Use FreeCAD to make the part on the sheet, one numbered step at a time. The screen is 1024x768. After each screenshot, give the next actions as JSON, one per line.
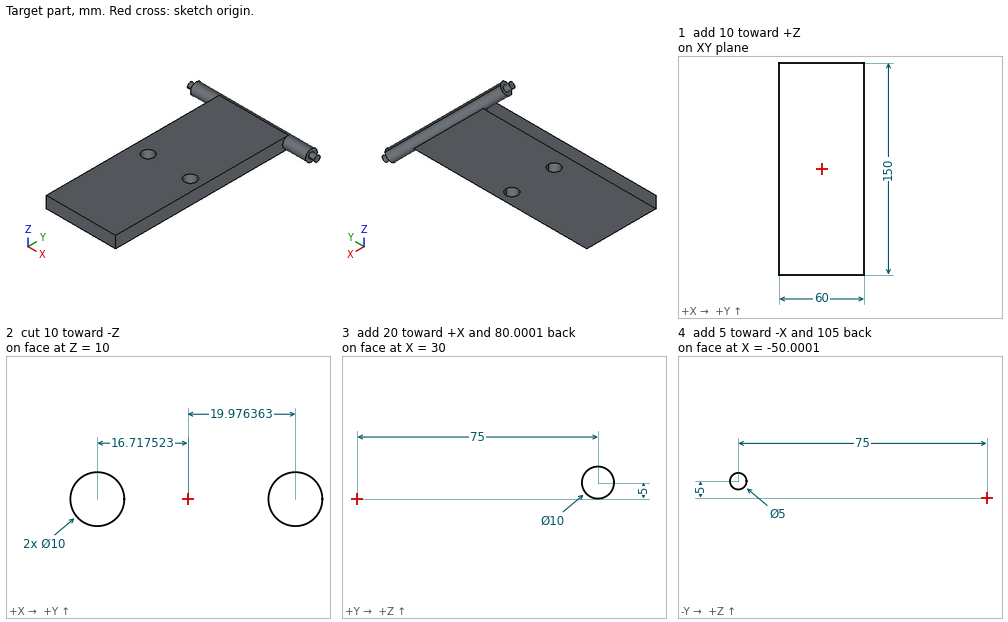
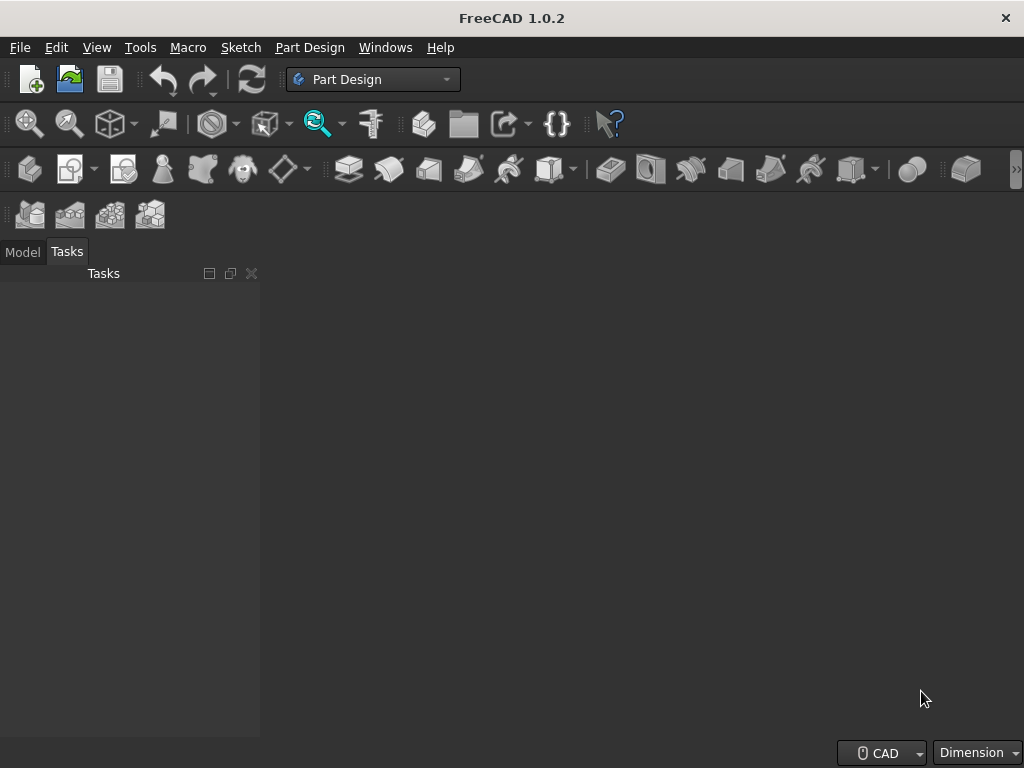
{"action": "left_click", "coordinate": [30, 80]}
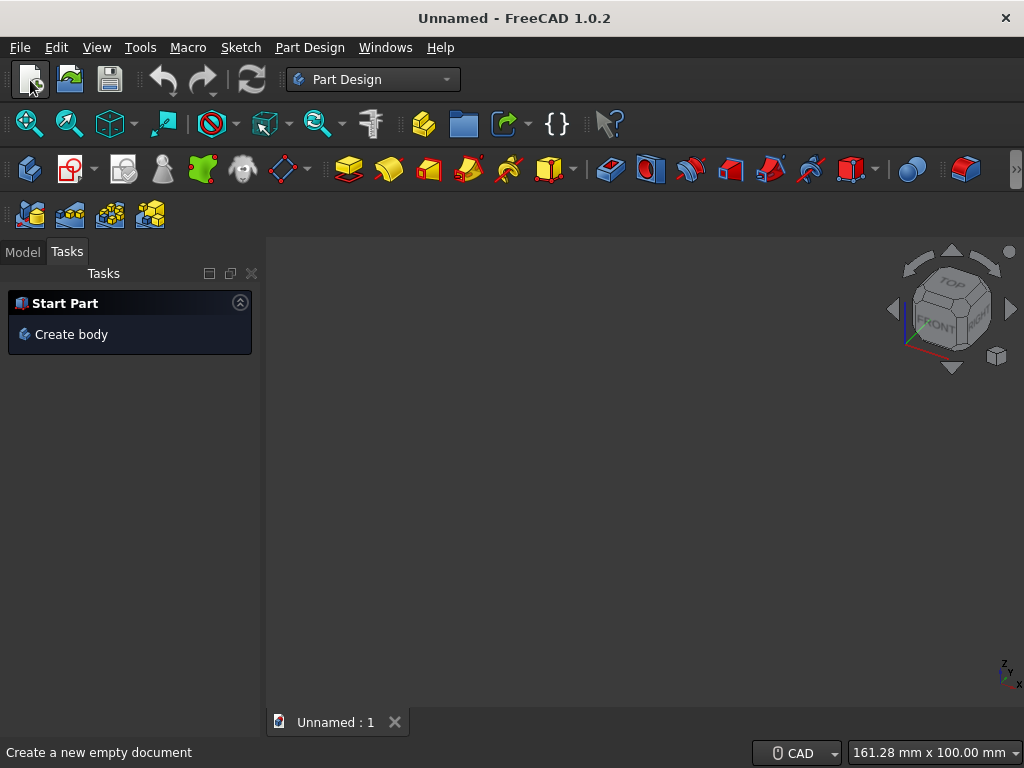
{"action": "left_click", "coordinate": [70, 170]}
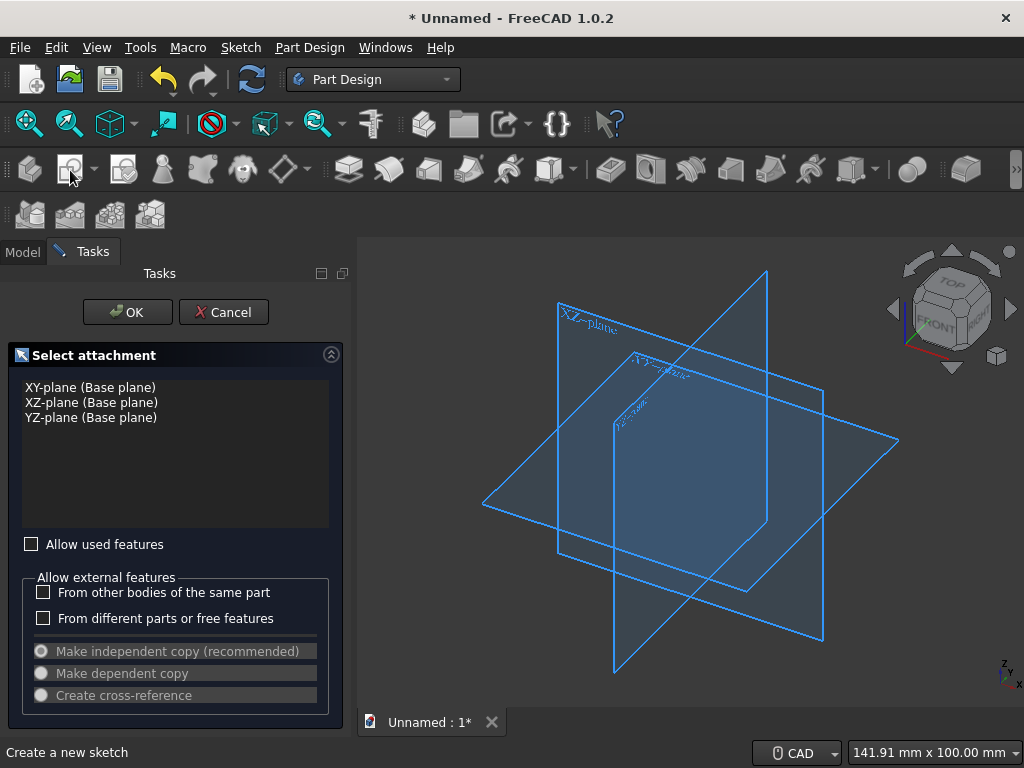
{"action": "left_click", "coordinate": [82, 388]}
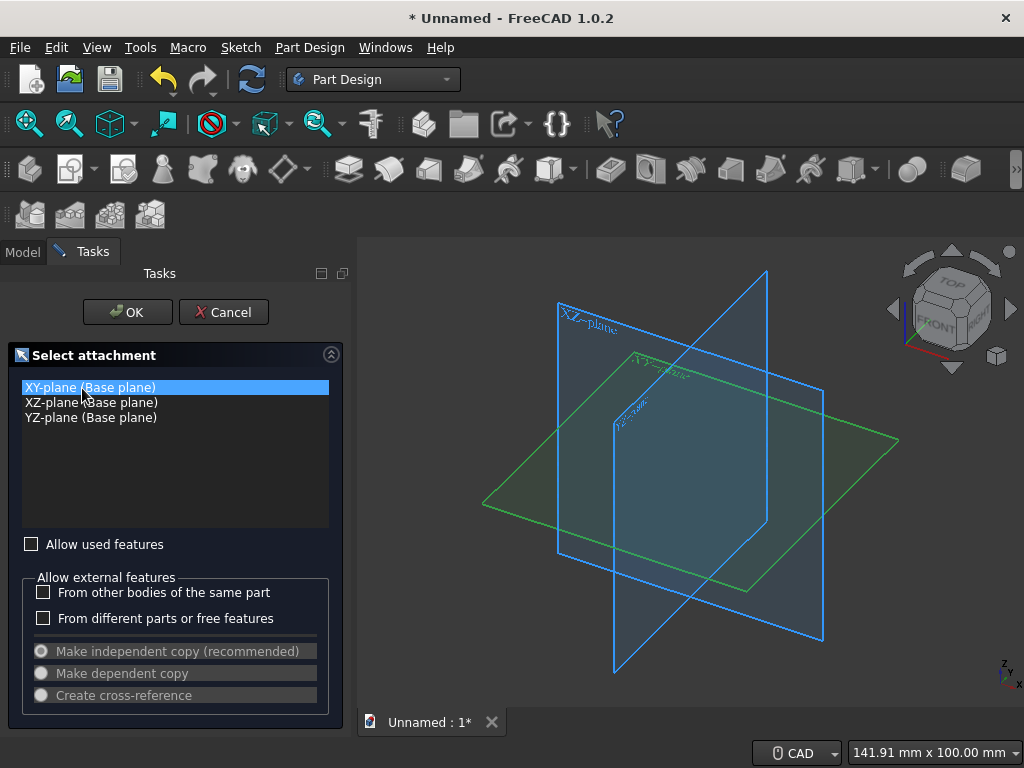
{"action": "left_click", "coordinate": [128, 312]}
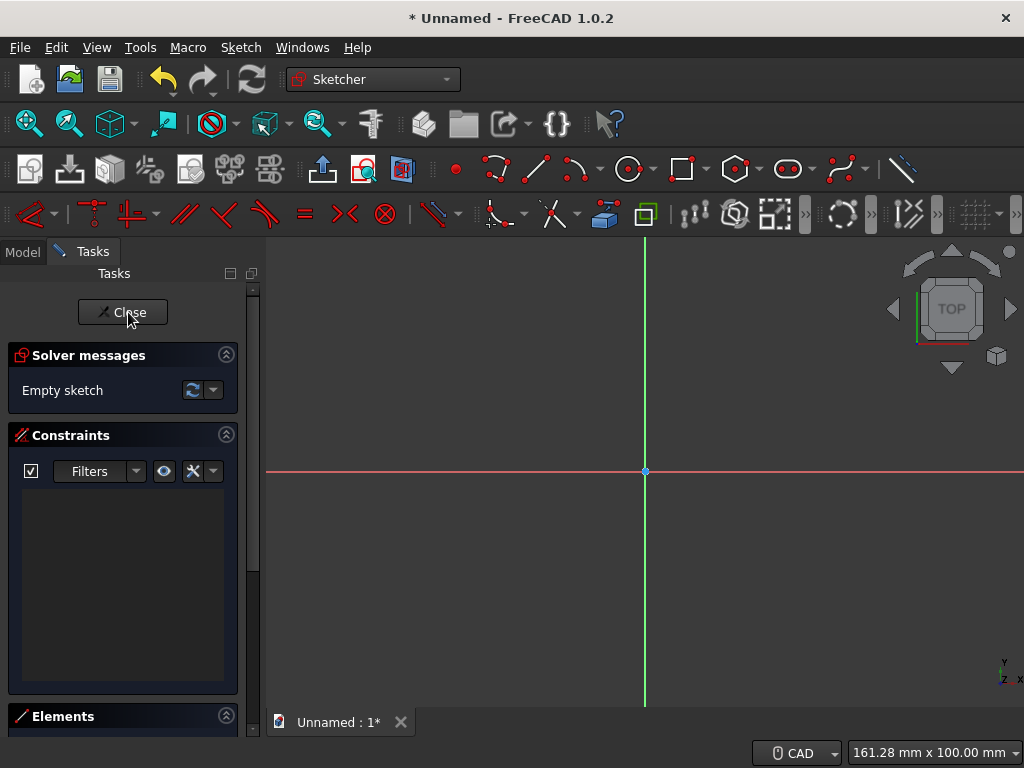
{"action": "scroll", "coordinate": [521, 472], "scroll_direction": "down", "scroll_amount": 4}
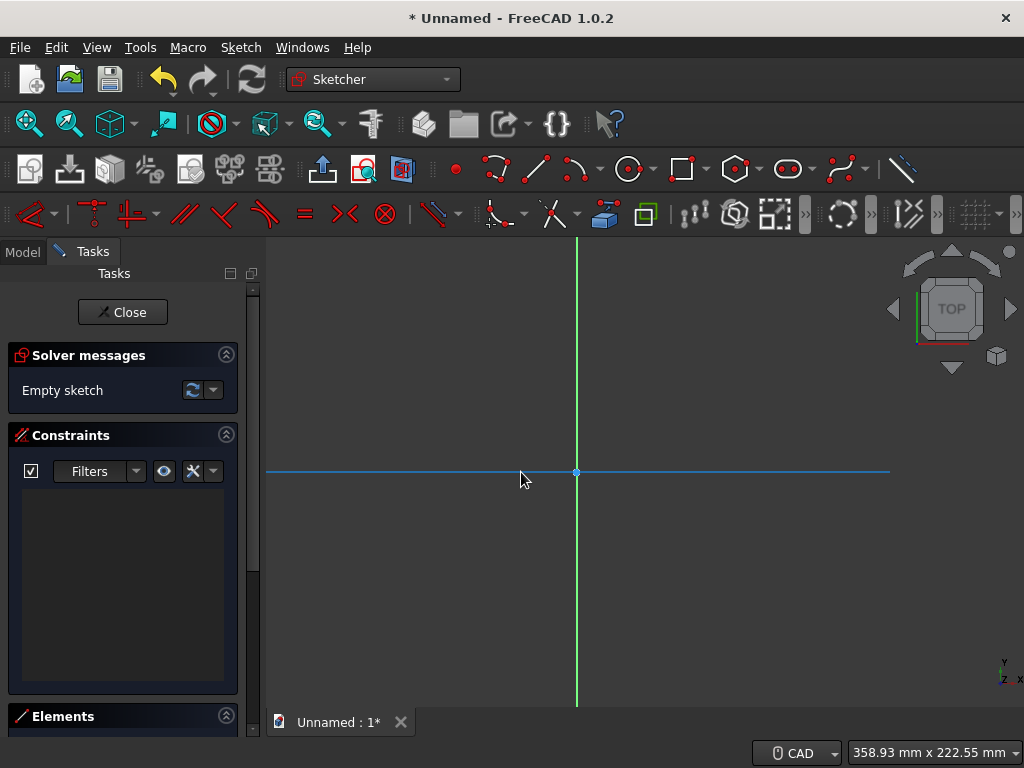
{"action": "left_click", "coordinate": [708, 170]}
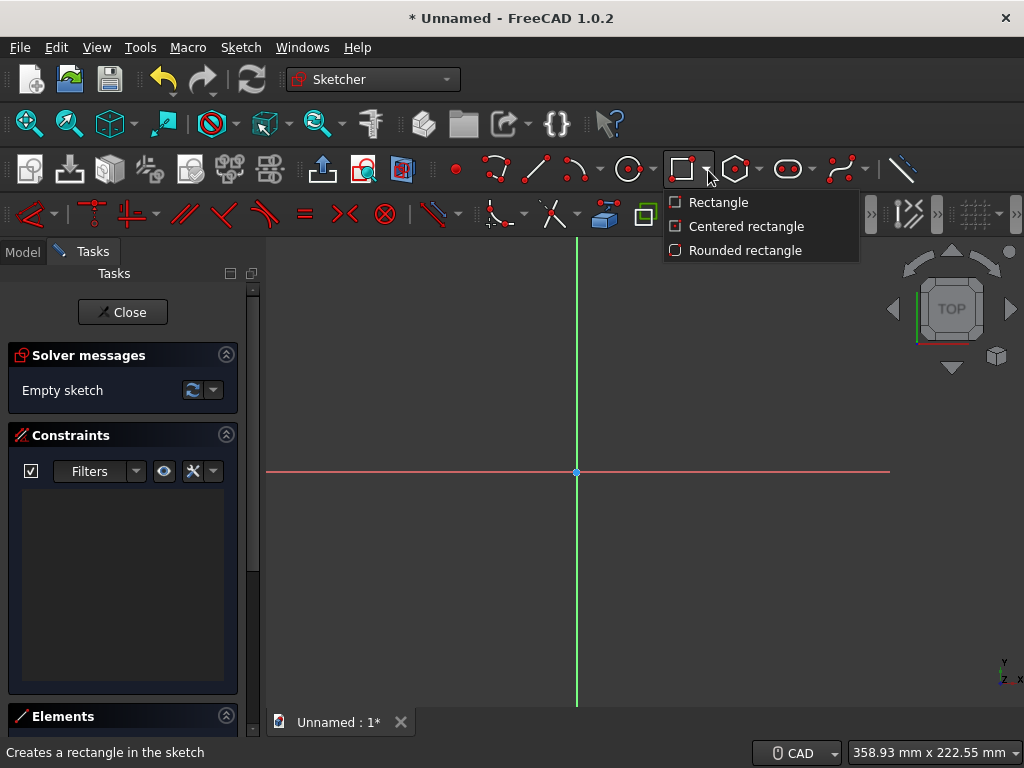
{"action": "left_click", "coordinate": [762, 226]}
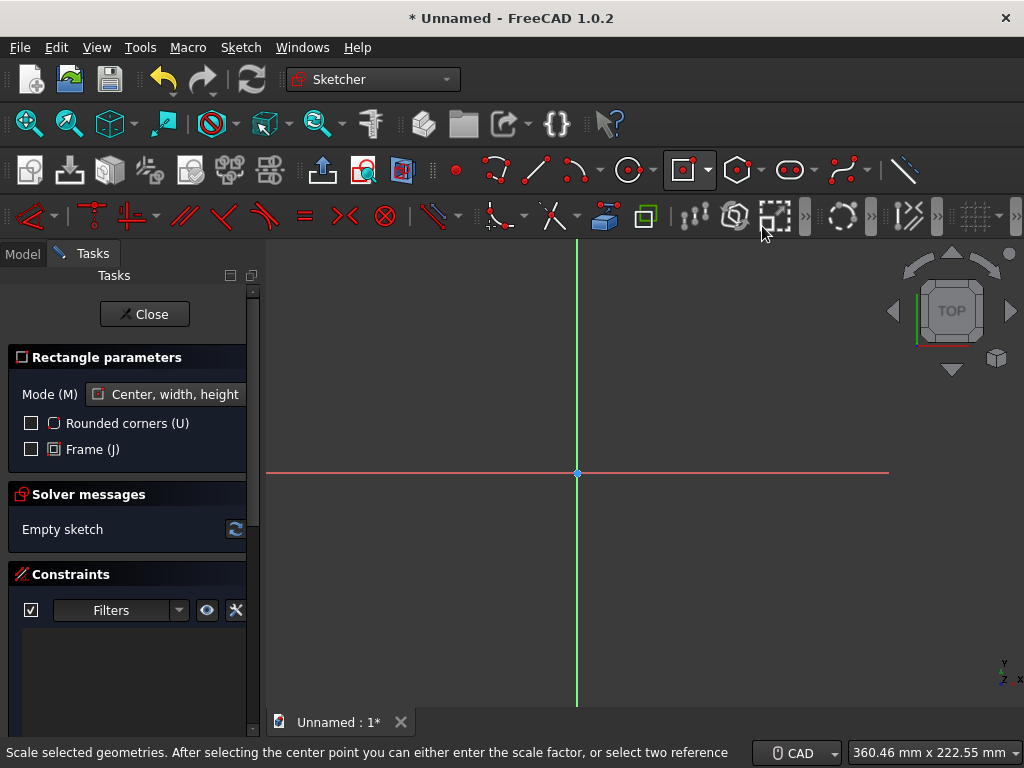
{"action": "left_click", "coordinate": [577, 473]}
{"action": "left_click", "coordinate": [640, 316]}
{"action": "key", "text": "Escape"}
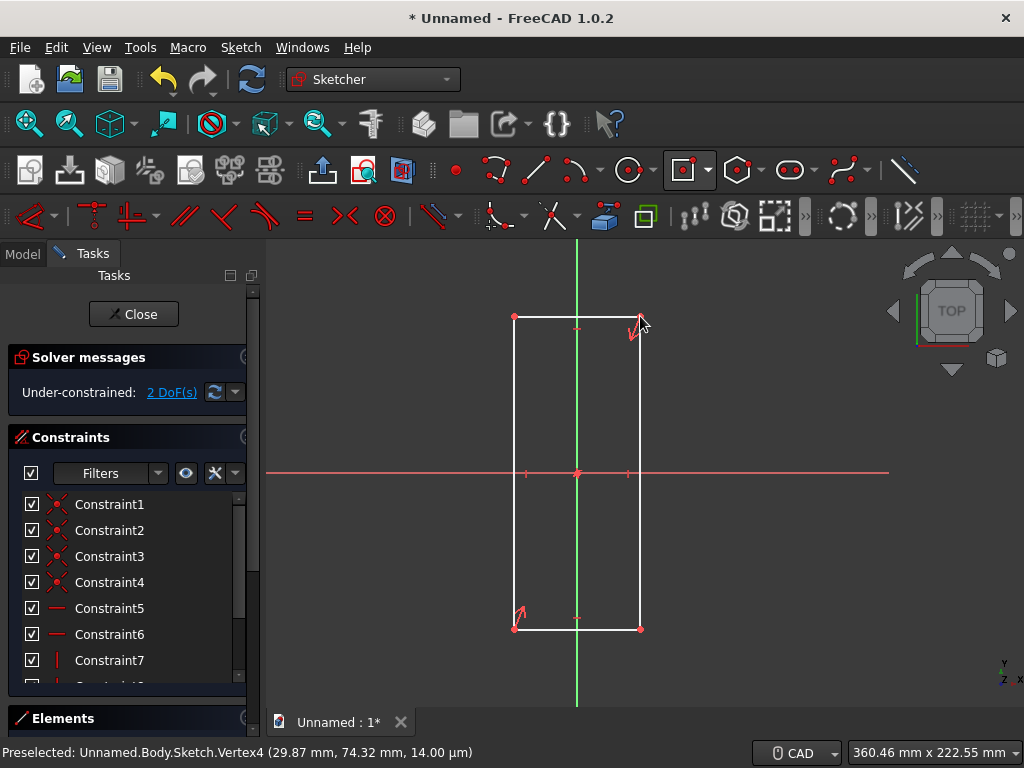
{"action": "left_click", "coordinate": [30, 216]}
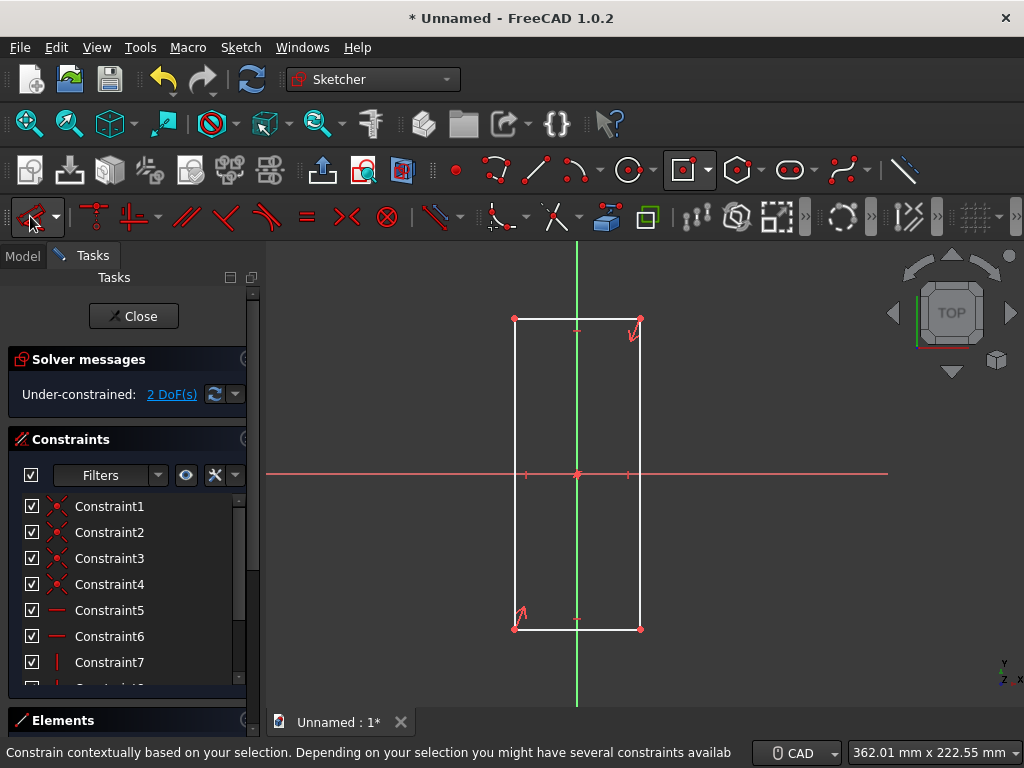
{"action": "left_click", "coordinate": [552, 630]}
{"action": "left_click", "coordinate": [549, 664]}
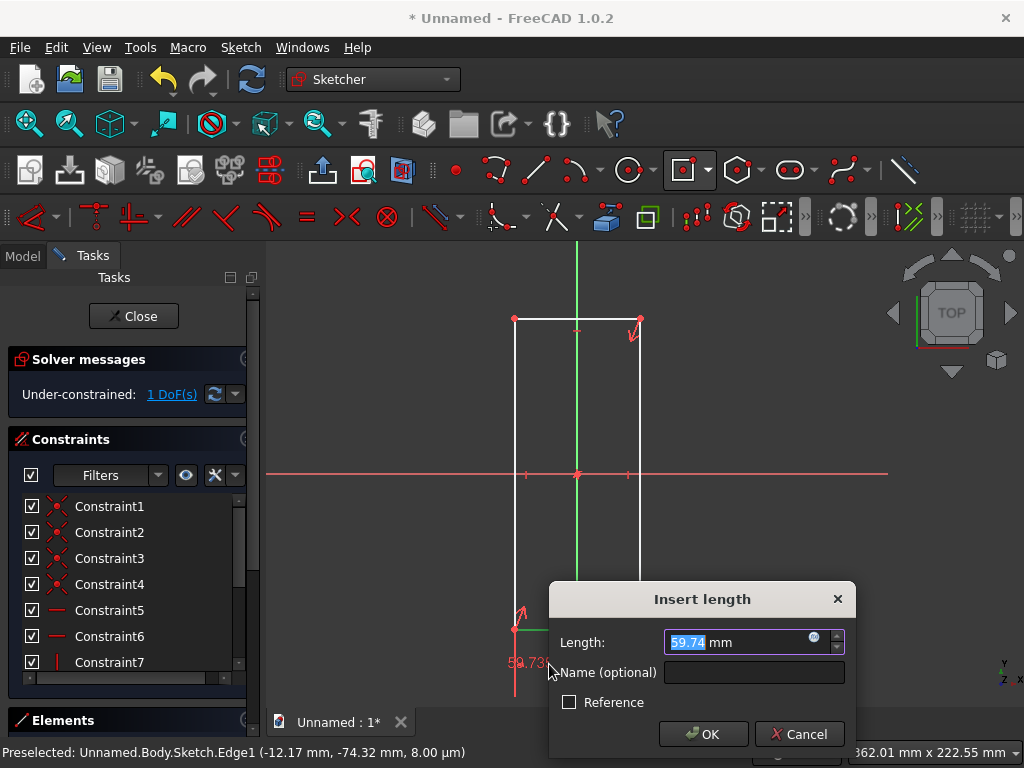
{"action": "type", "text": "60"}
{"action": "key", "text": "Return"}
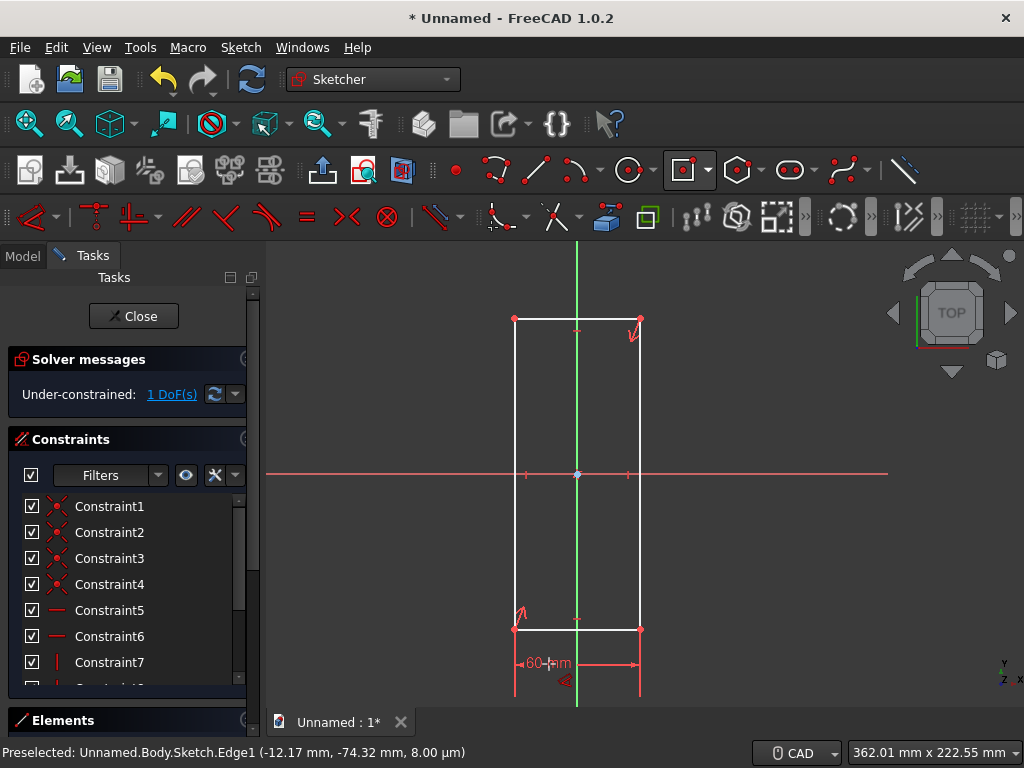
{"action": "left_click", "coordinate": [640, 537]}
{"action": "left_click", "coordinate": [674, 403]}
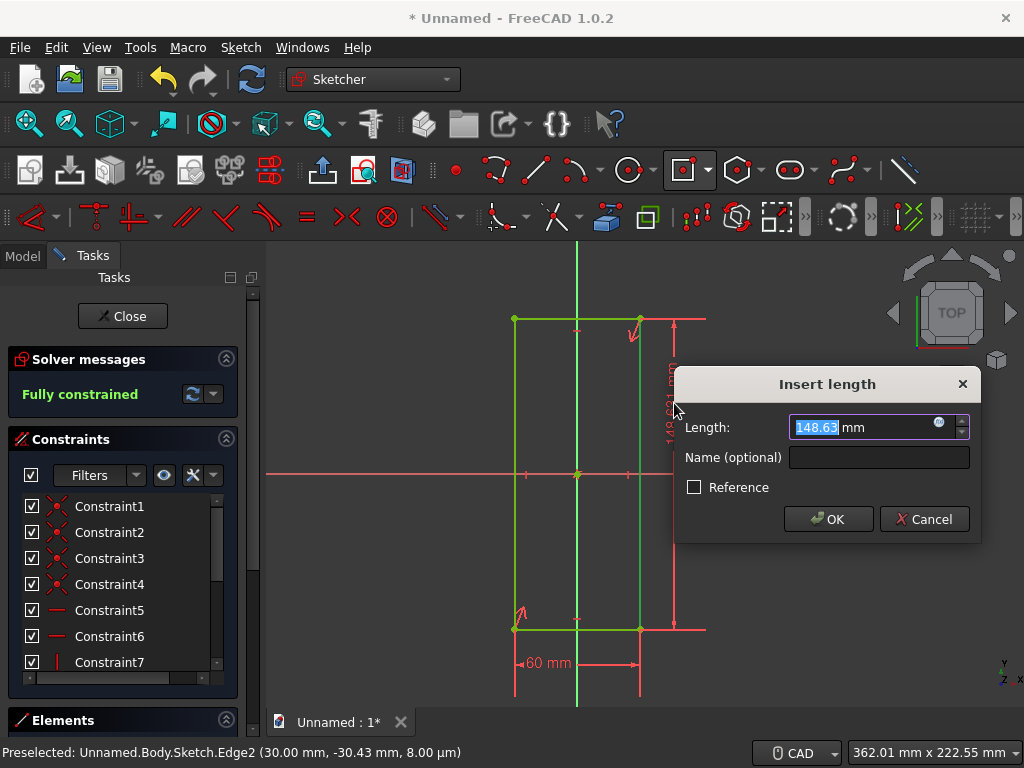
{"action": "type", "text": "150"}
{"action": "key", "text": "Return"}
{"action": "key", "text": "Escape"}